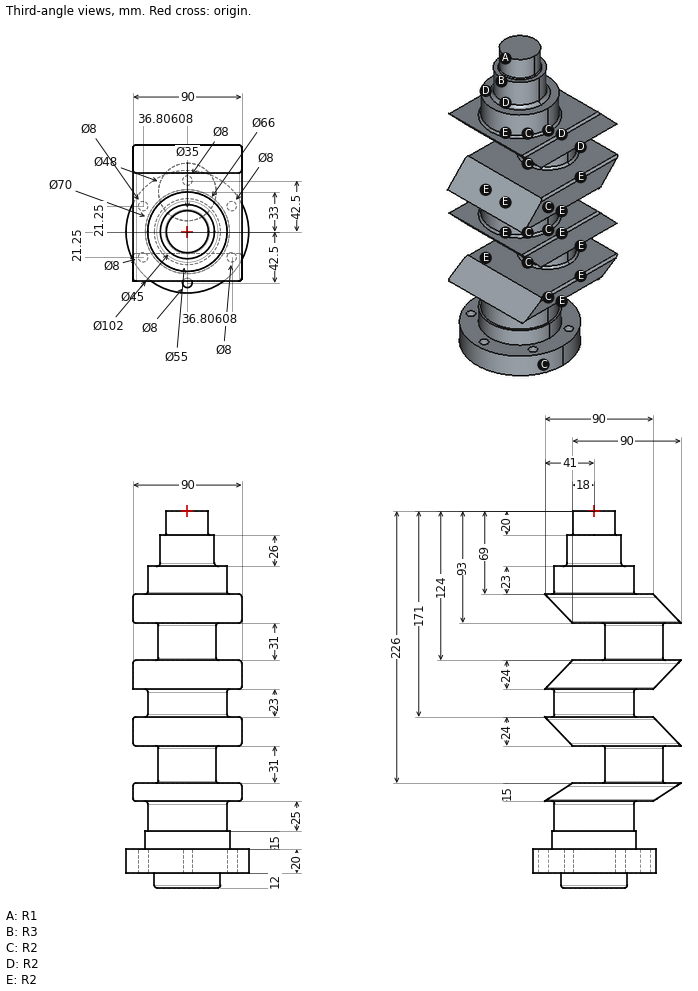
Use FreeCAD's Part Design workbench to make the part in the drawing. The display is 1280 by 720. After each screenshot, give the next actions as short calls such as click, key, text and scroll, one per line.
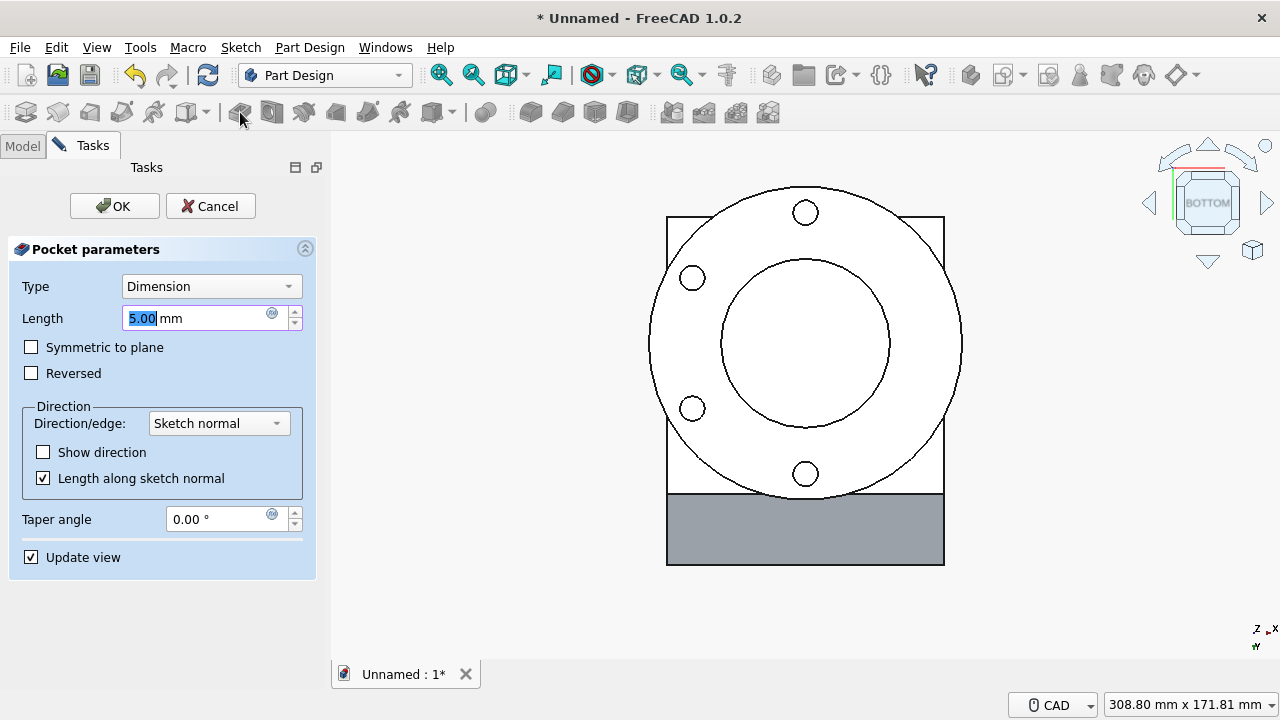
click(212, 286)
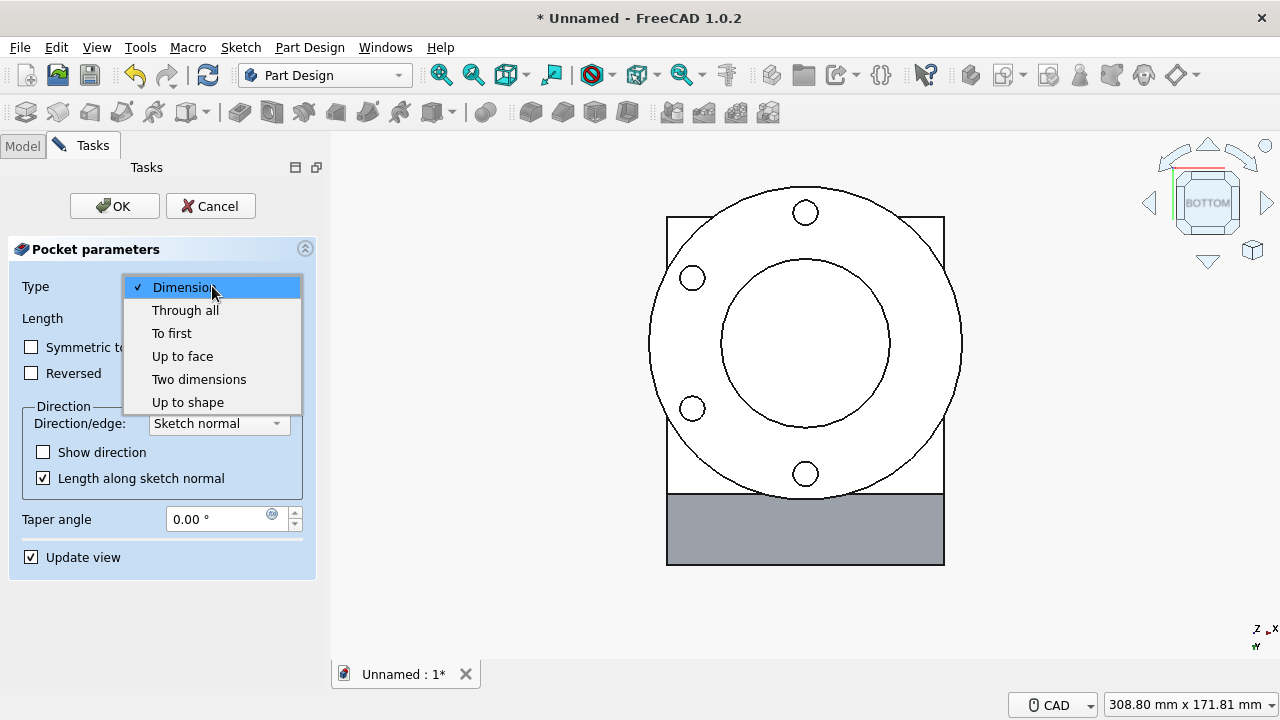
click(212, 334)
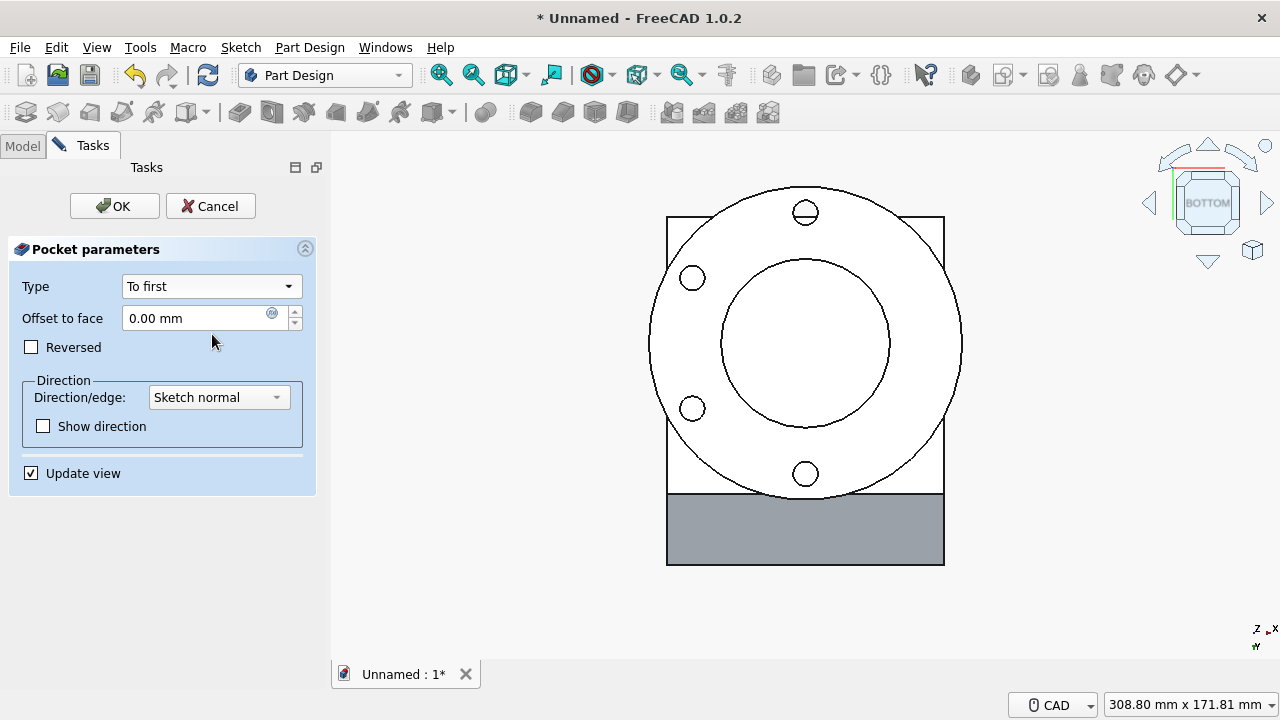
click(115, 206)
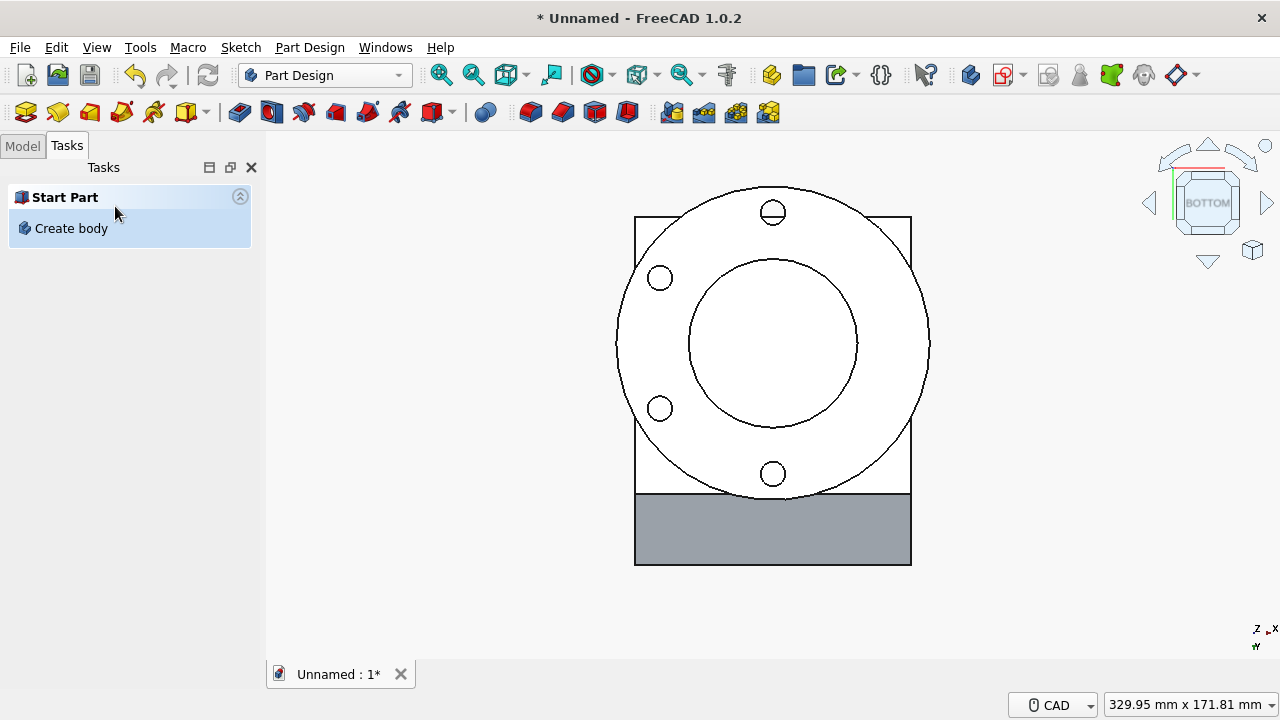
click(863, 432)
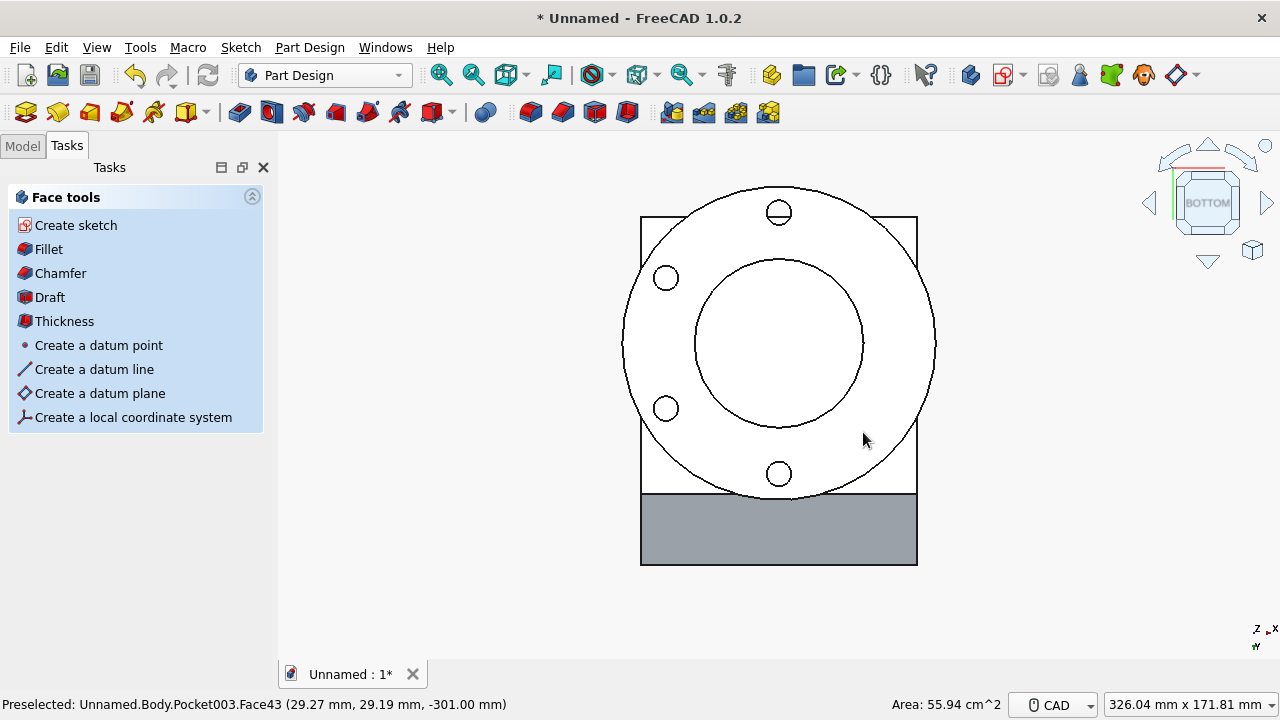
click(1004, 76)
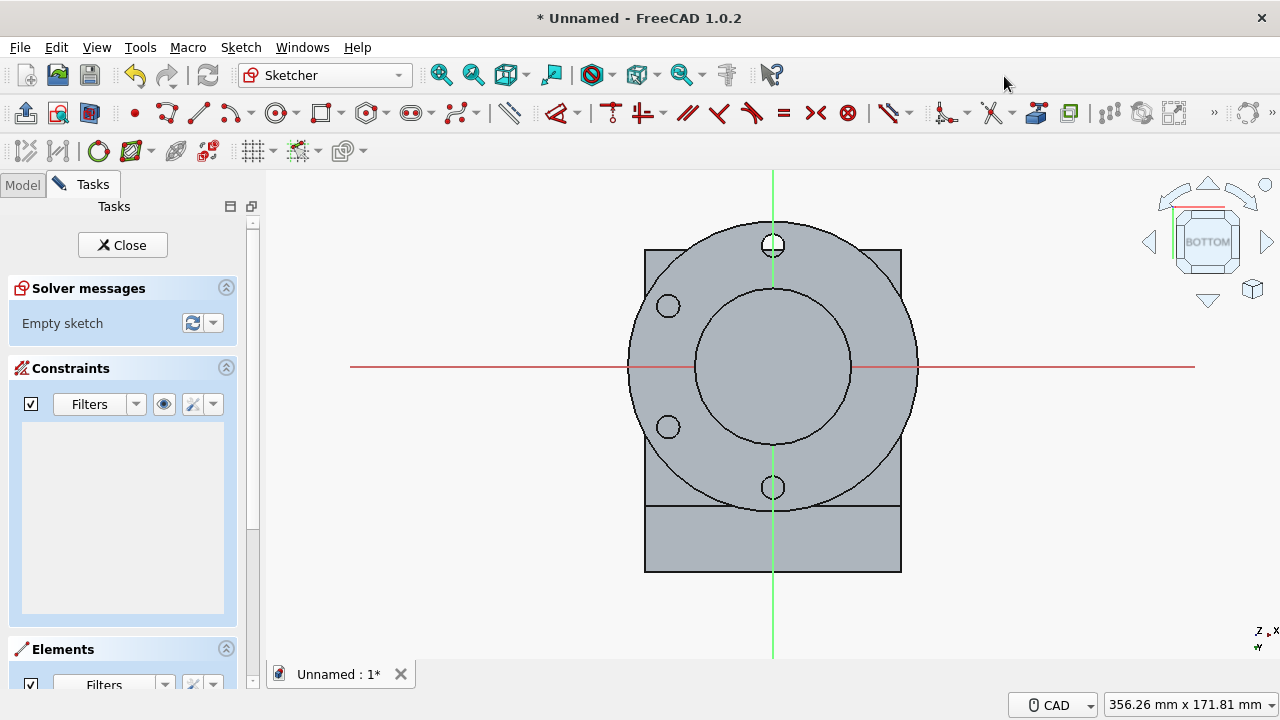
click(90, 114)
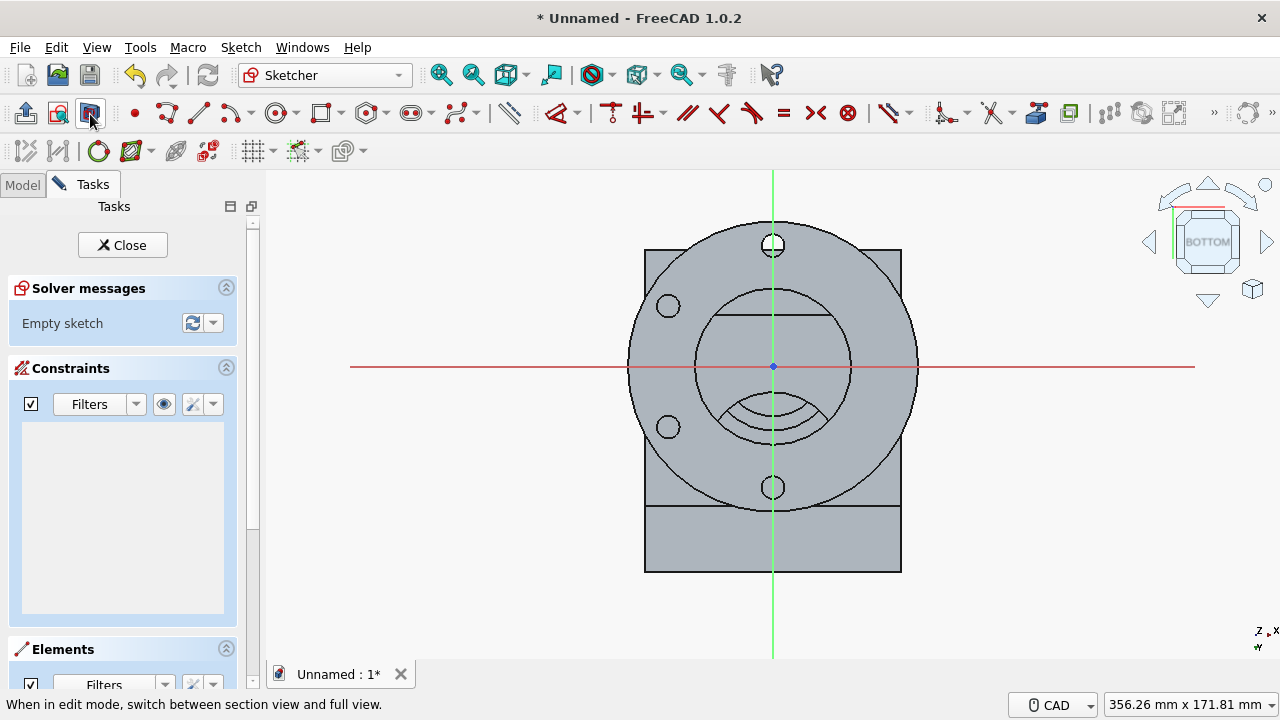
scroll(892, 297, up, 13)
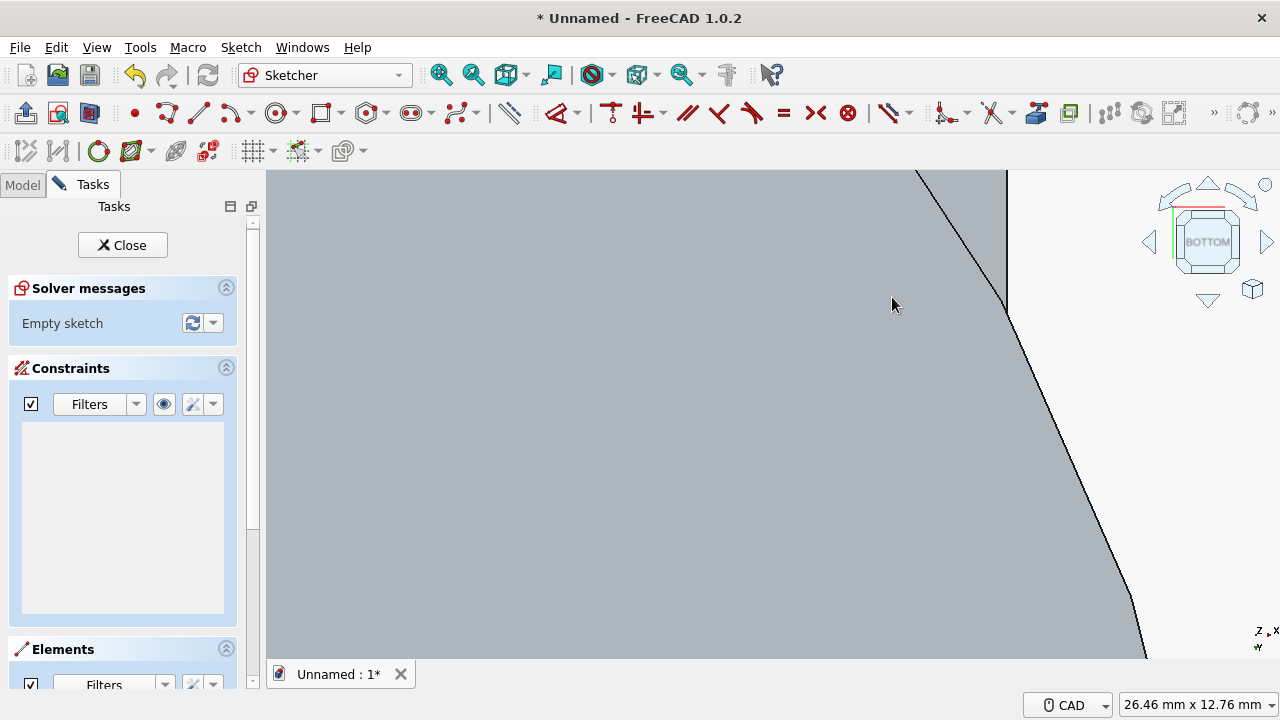
click(276, 114)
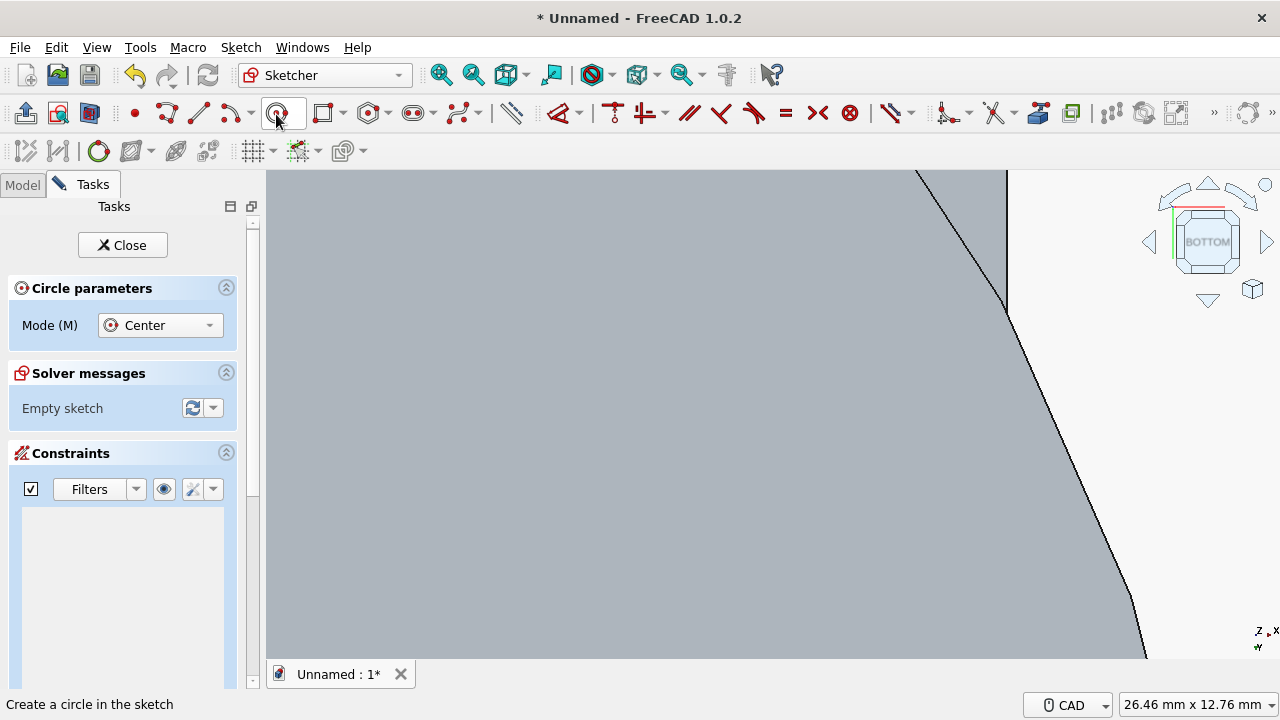
click(693, 417)
move(801, 308)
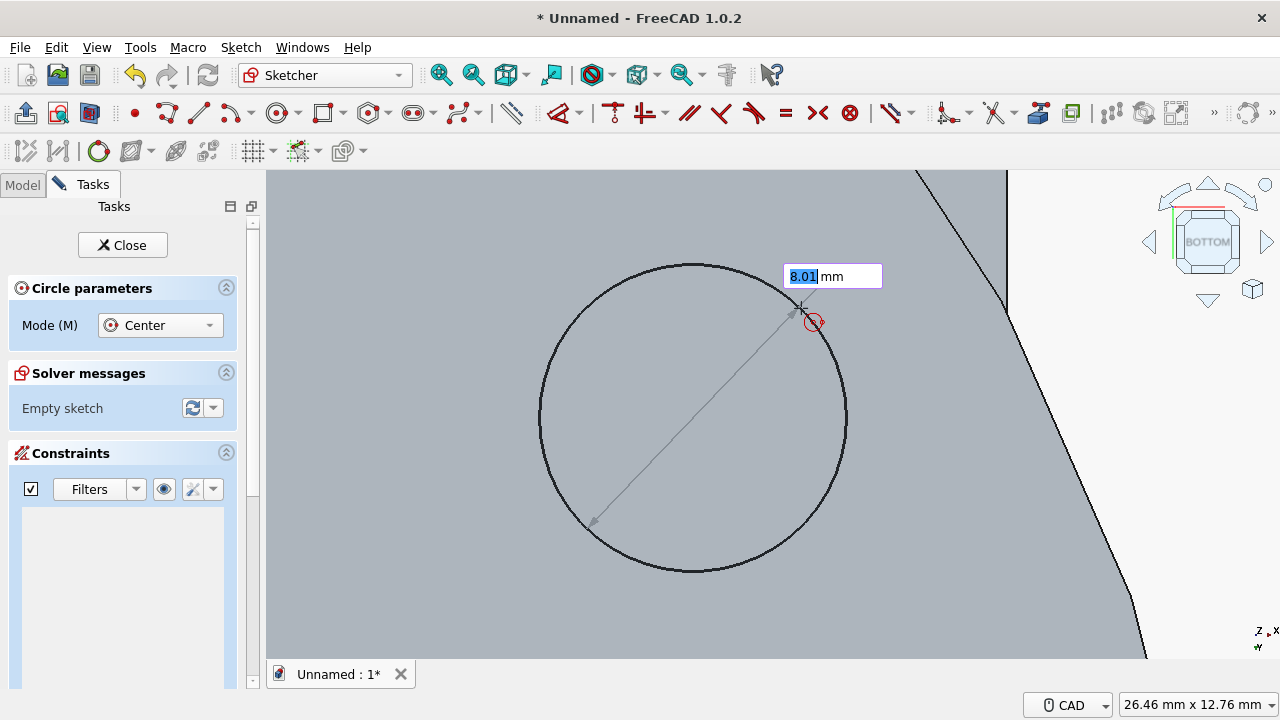
text(8)
key(Return)
key(Escape)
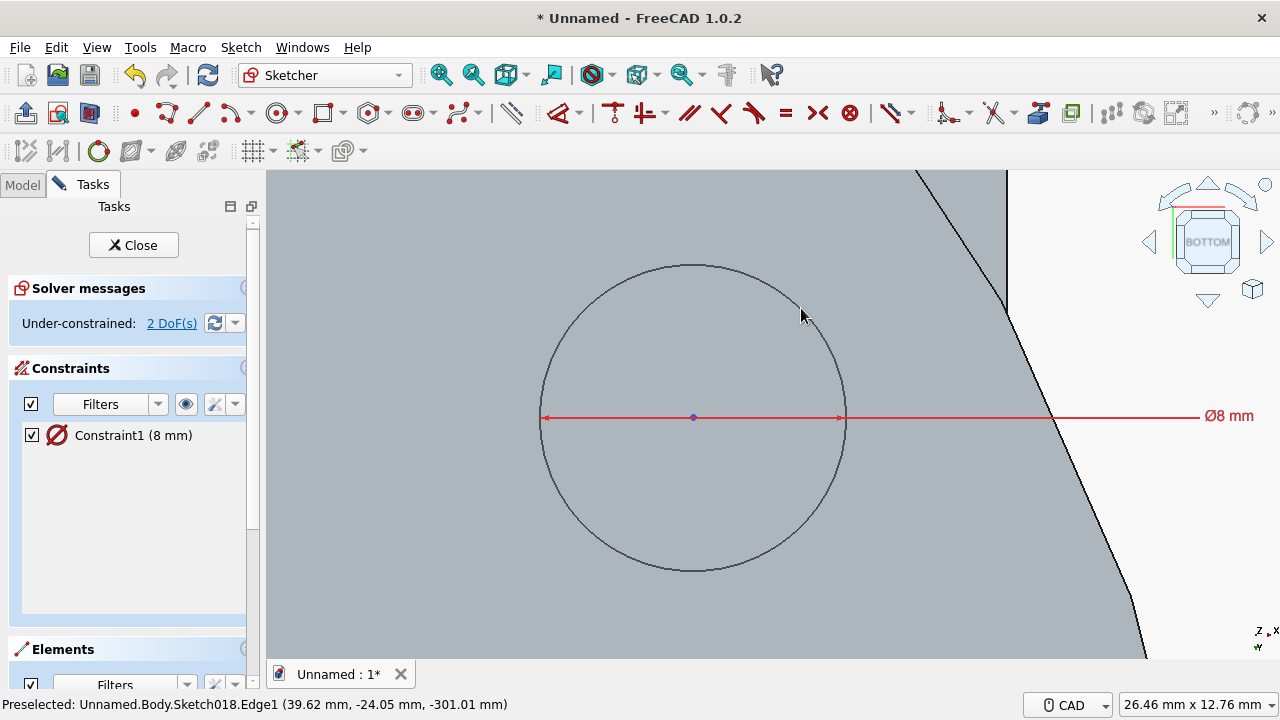
click(558, 114)